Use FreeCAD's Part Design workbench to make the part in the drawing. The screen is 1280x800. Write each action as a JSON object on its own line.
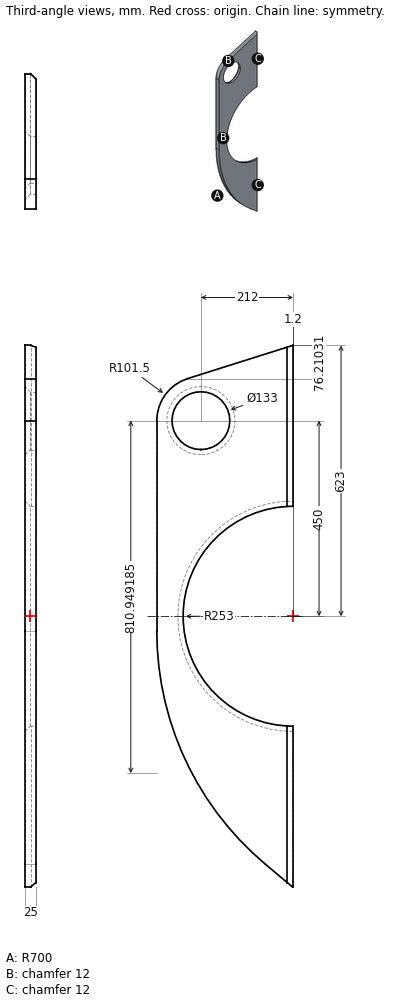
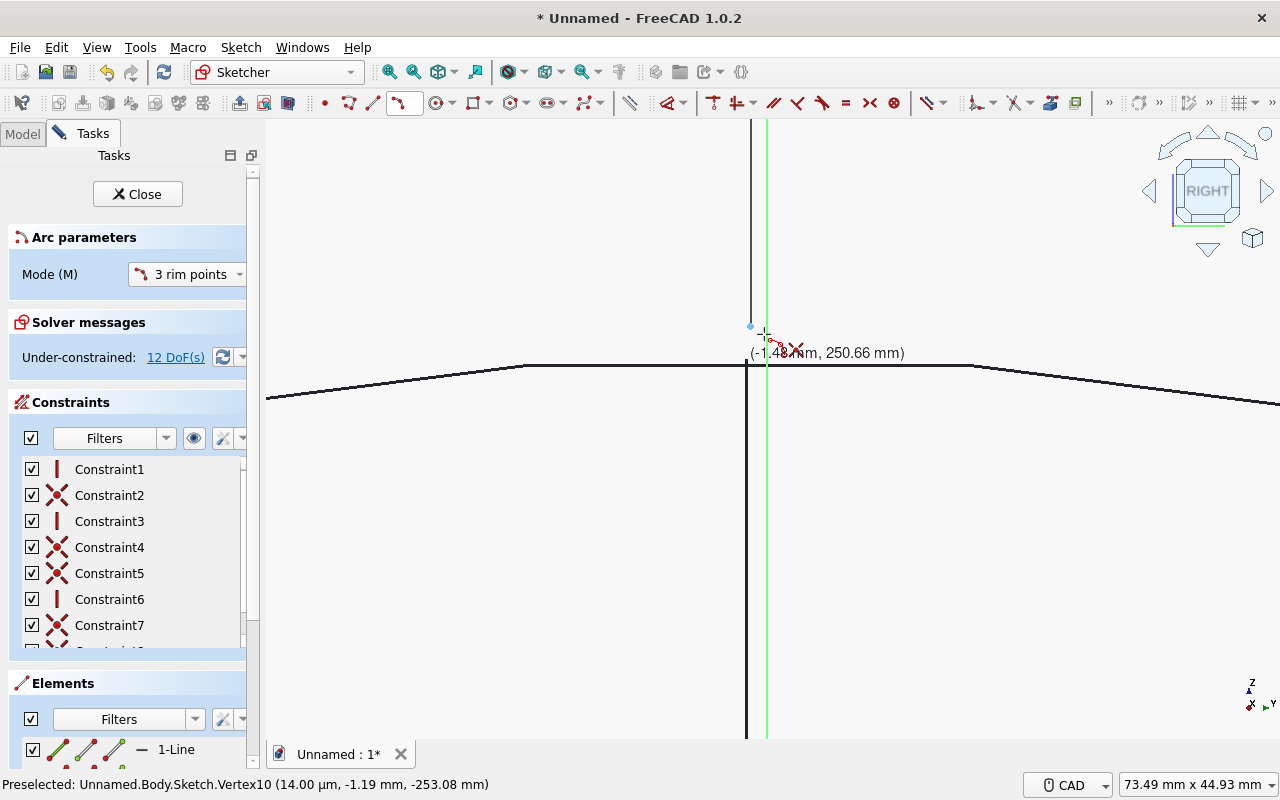
{"action": "left_click", "coordinate": [751, 327]}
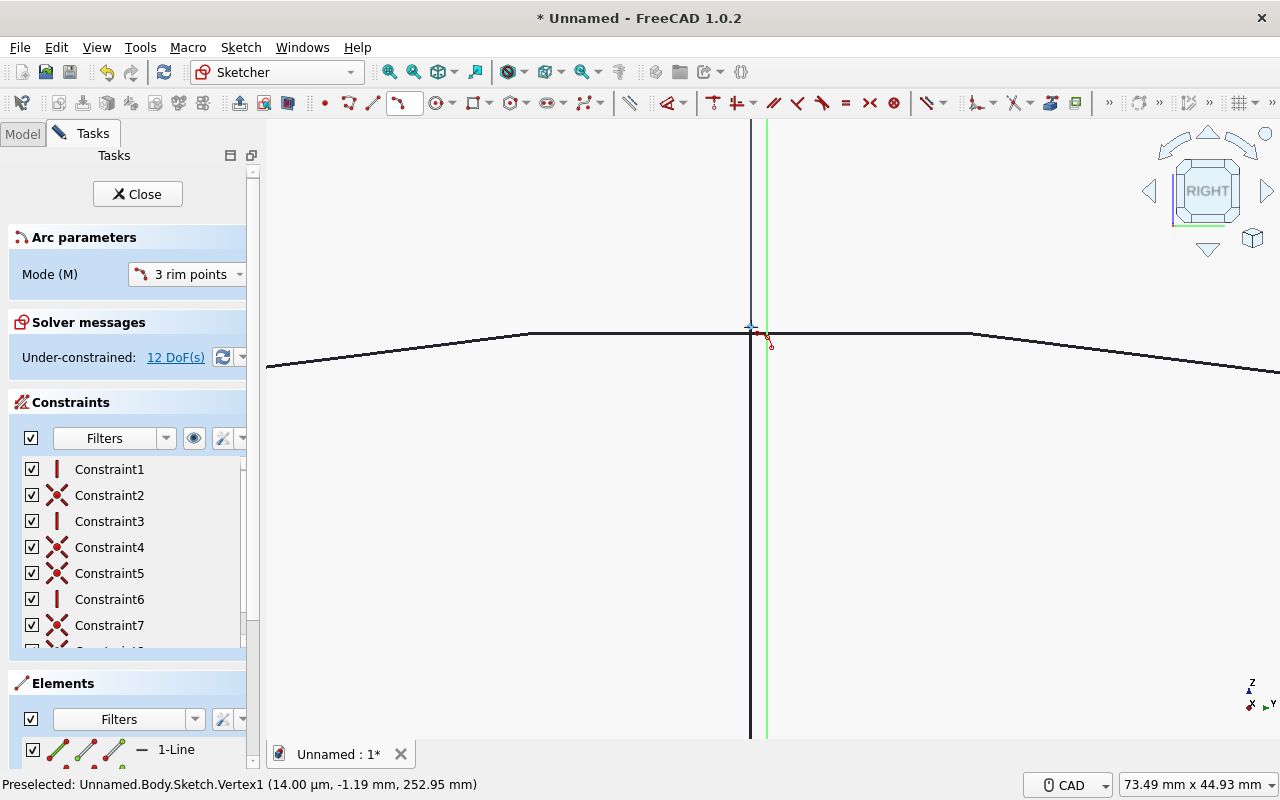
{"action": "scroll", "coordinate": [764, 334], "scroll_direction": "down", "scroll_amount": 18}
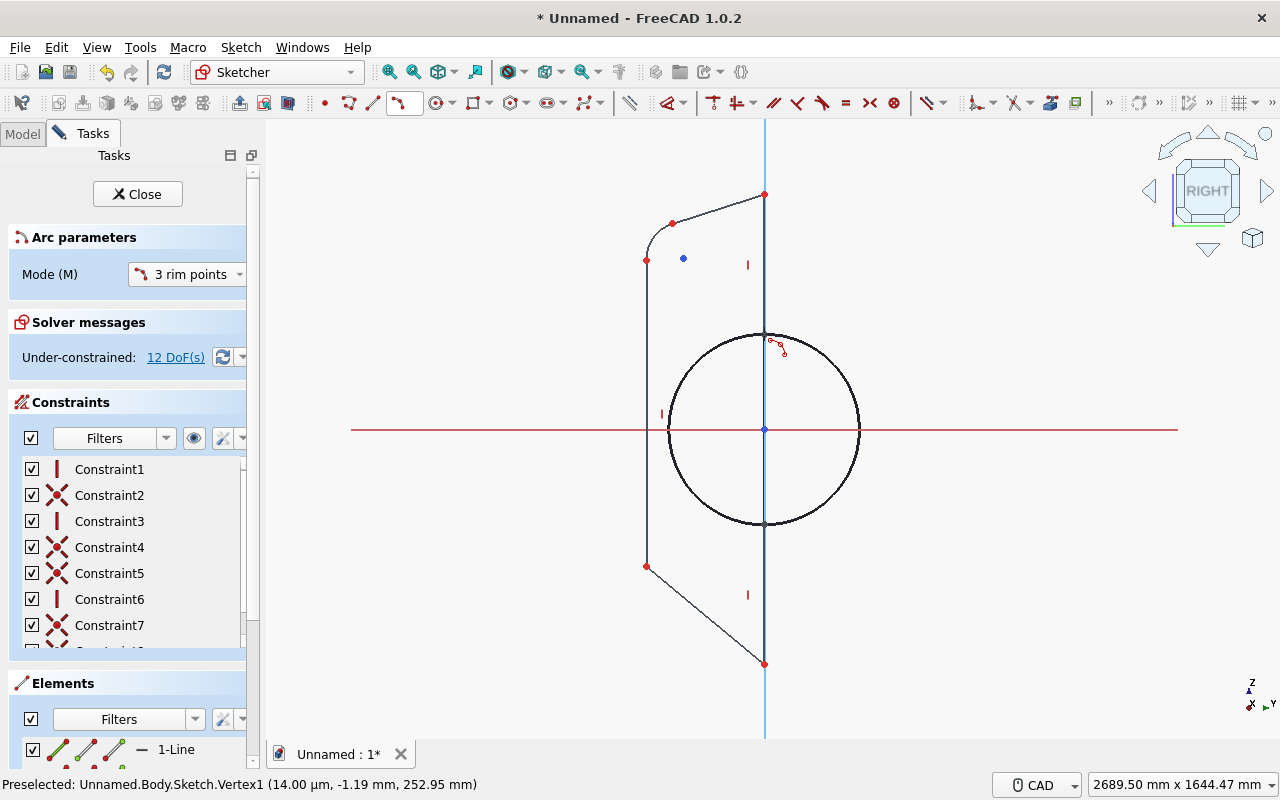
{"action": "left_click", "coordinate": [674, 400]}
{"action": "key", "text": "Escape"}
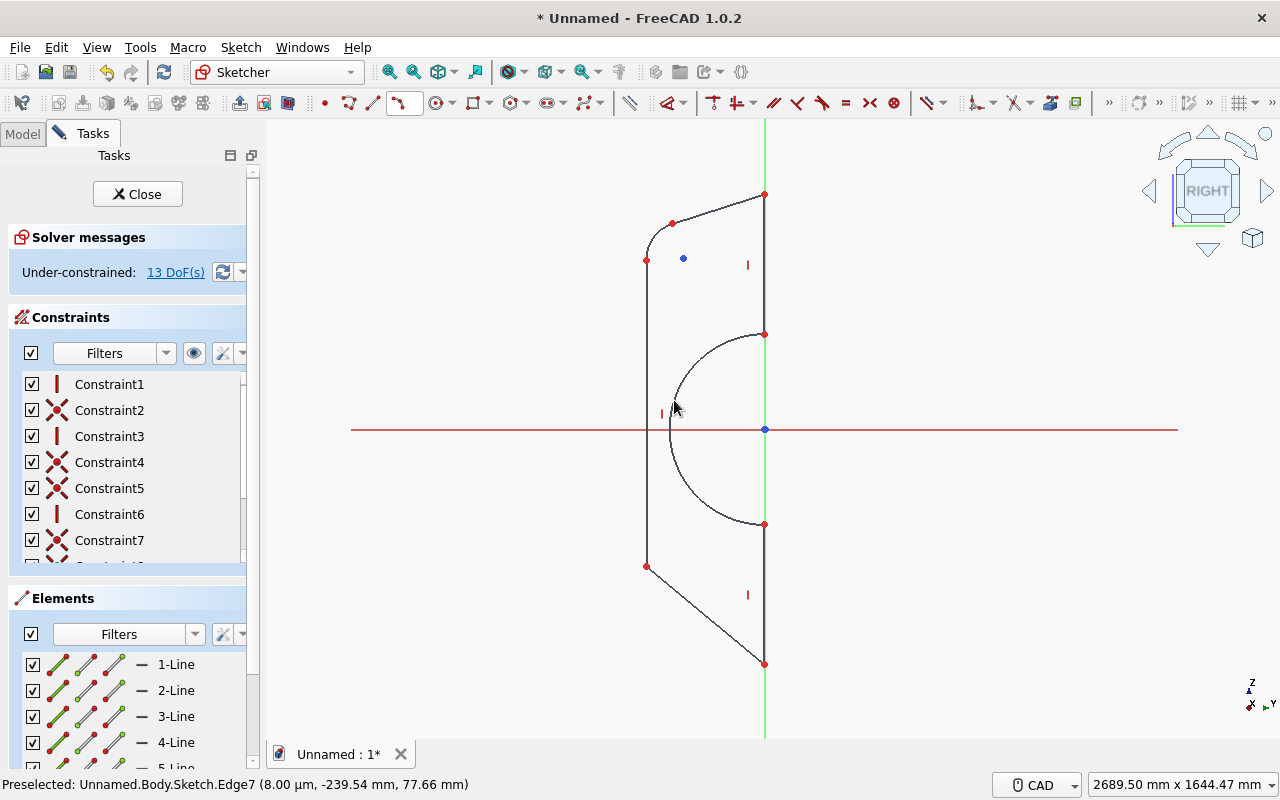
{"action": "left_click_drag", "start_coordinate": [755, 420], "coordinate": [775, 440]}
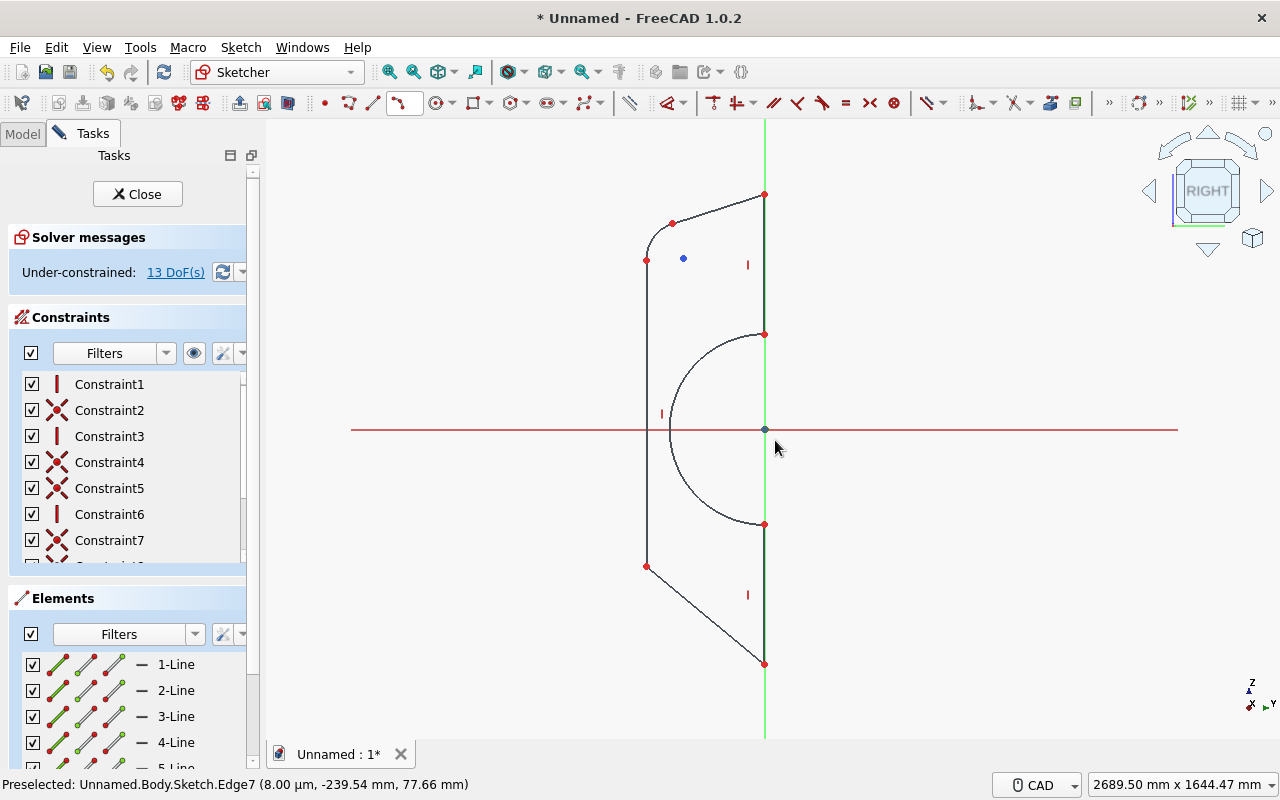
{"action": "left_click", "coordinate": [714, 104]}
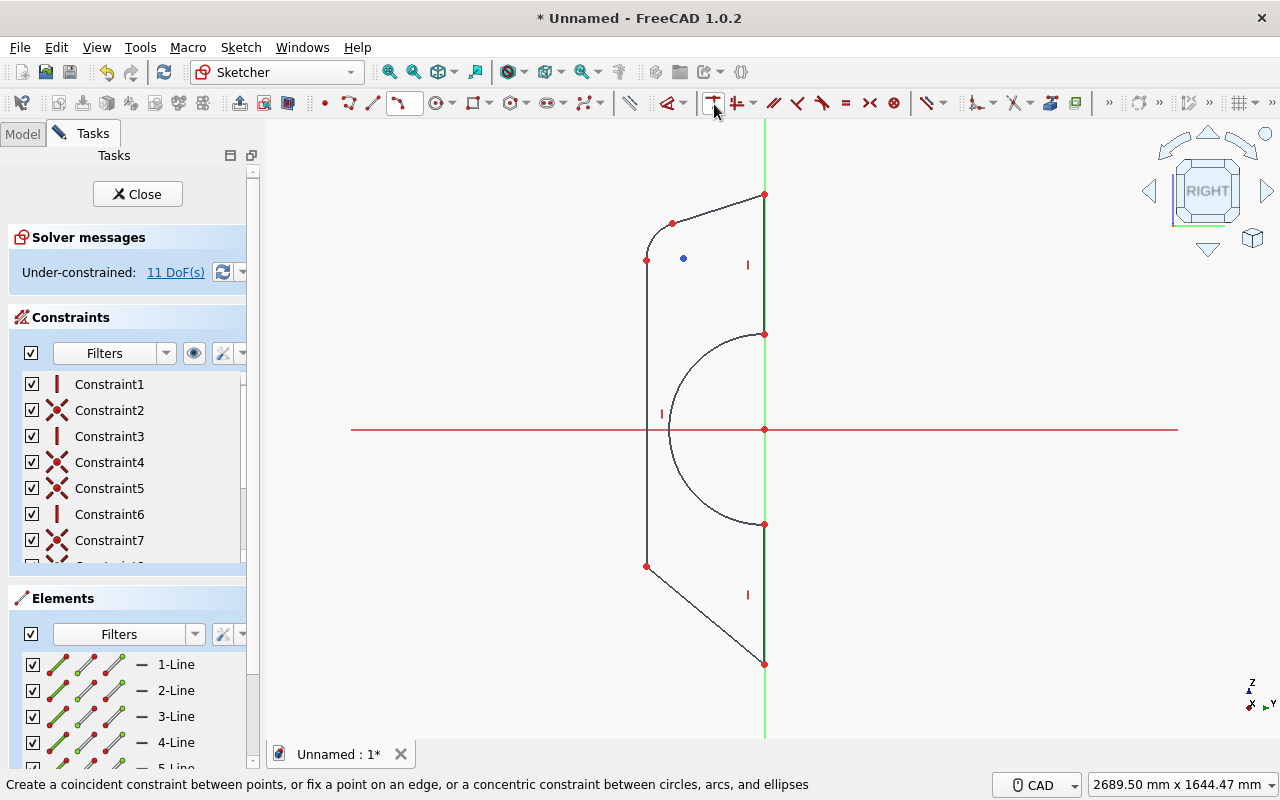
{"action": "left_click", "coordinate": [764, 195]}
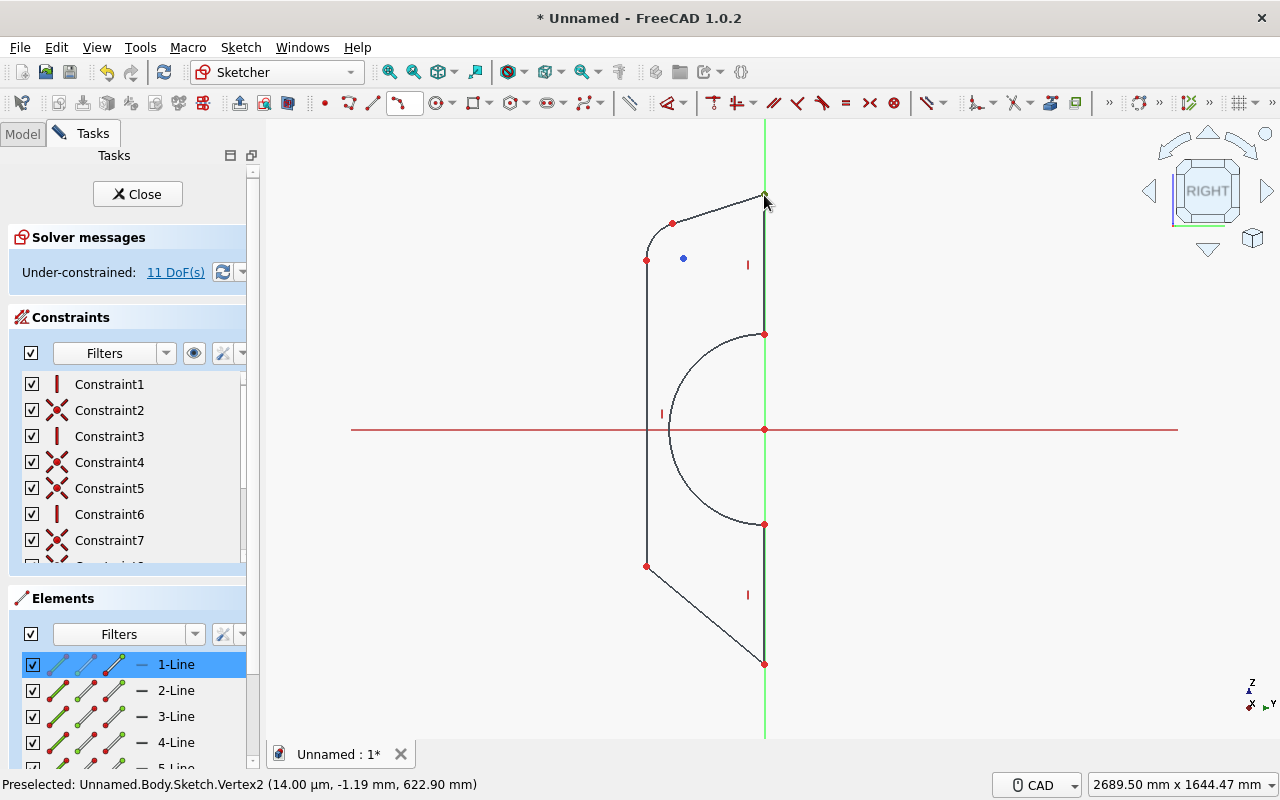
{"action": "left_click", "coordinate": [764, 664]}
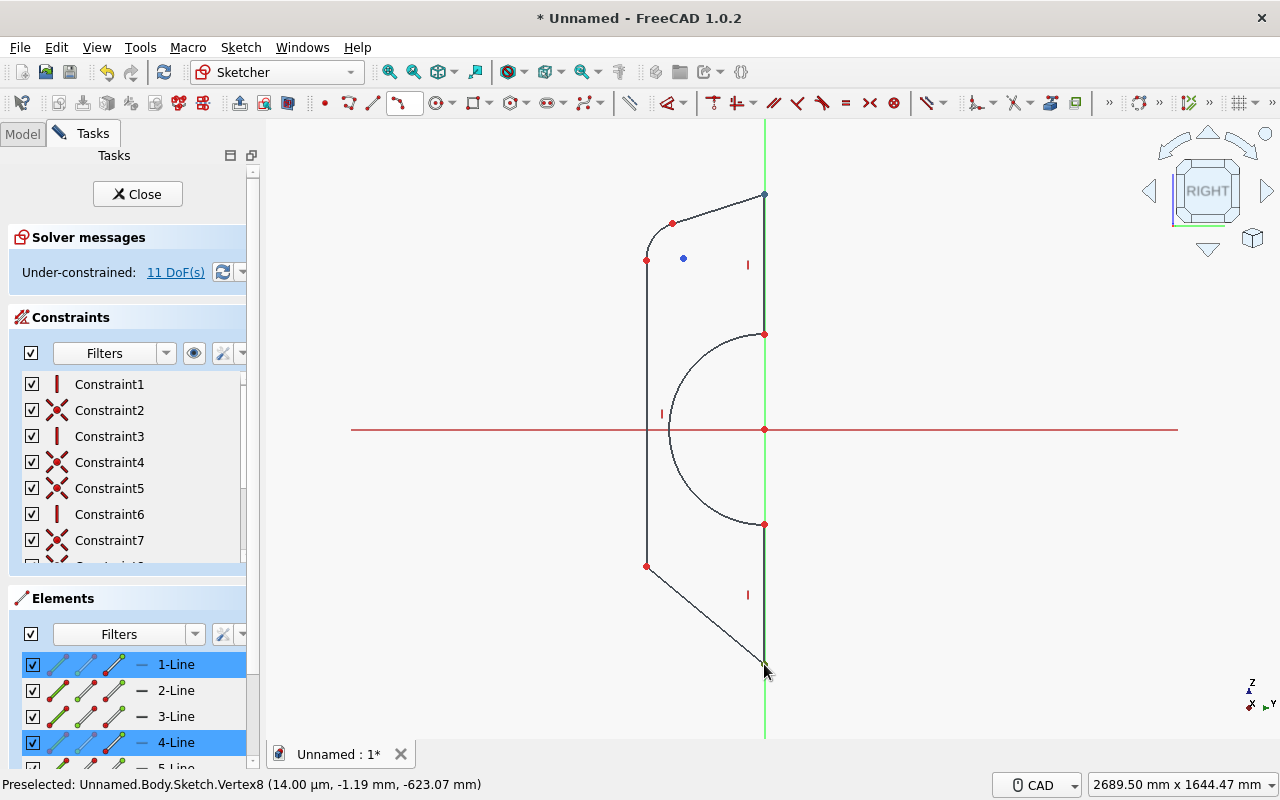
{"action": "left_click", "coordinate": [353, 430]}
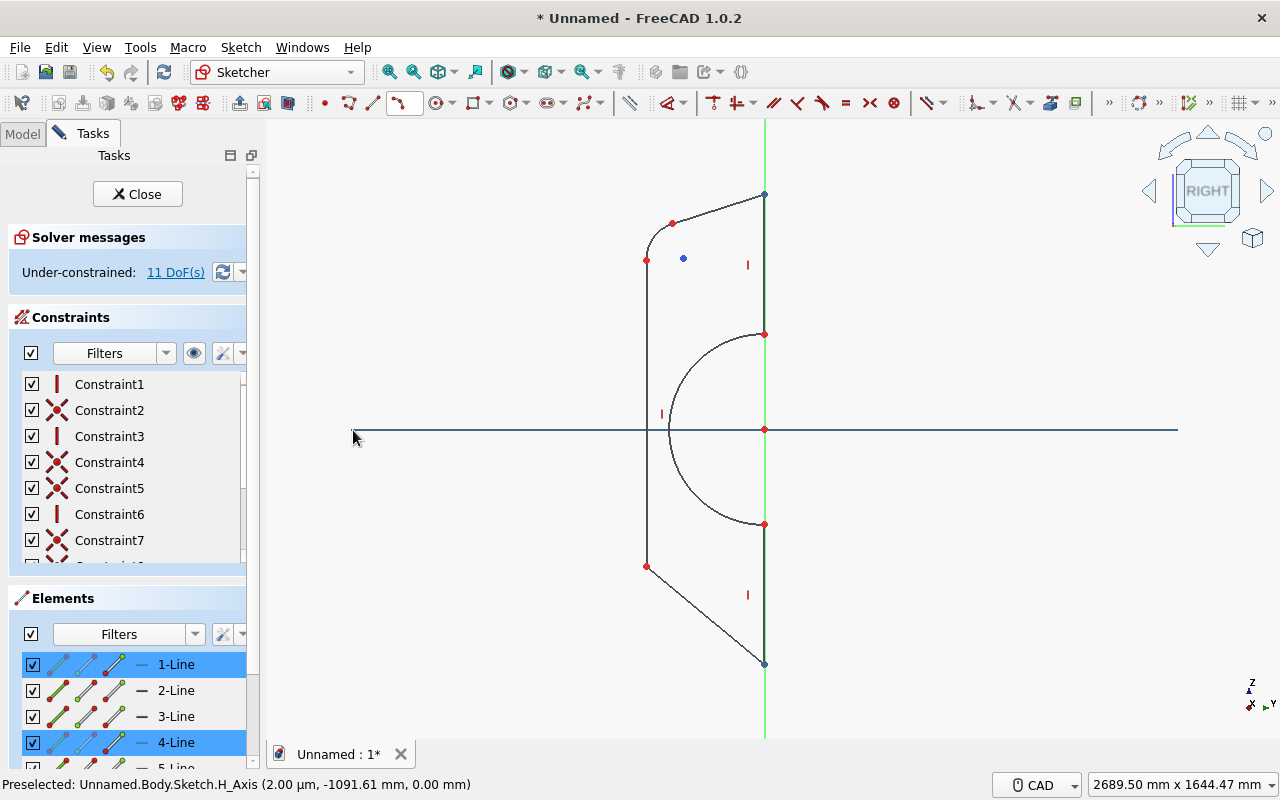
{"action": "left_click", "coordinate": [870, 104]}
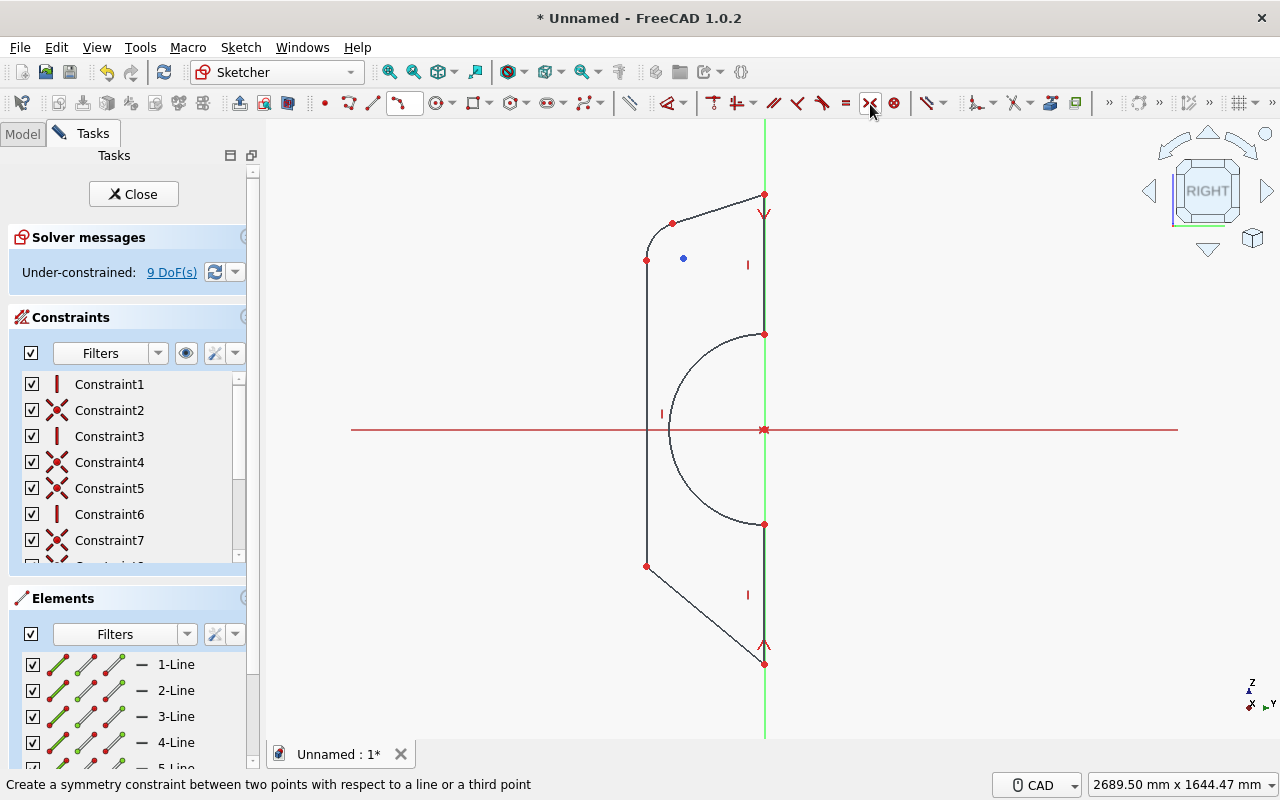
{"action": "left_click", "coordinate": [668, 104]}